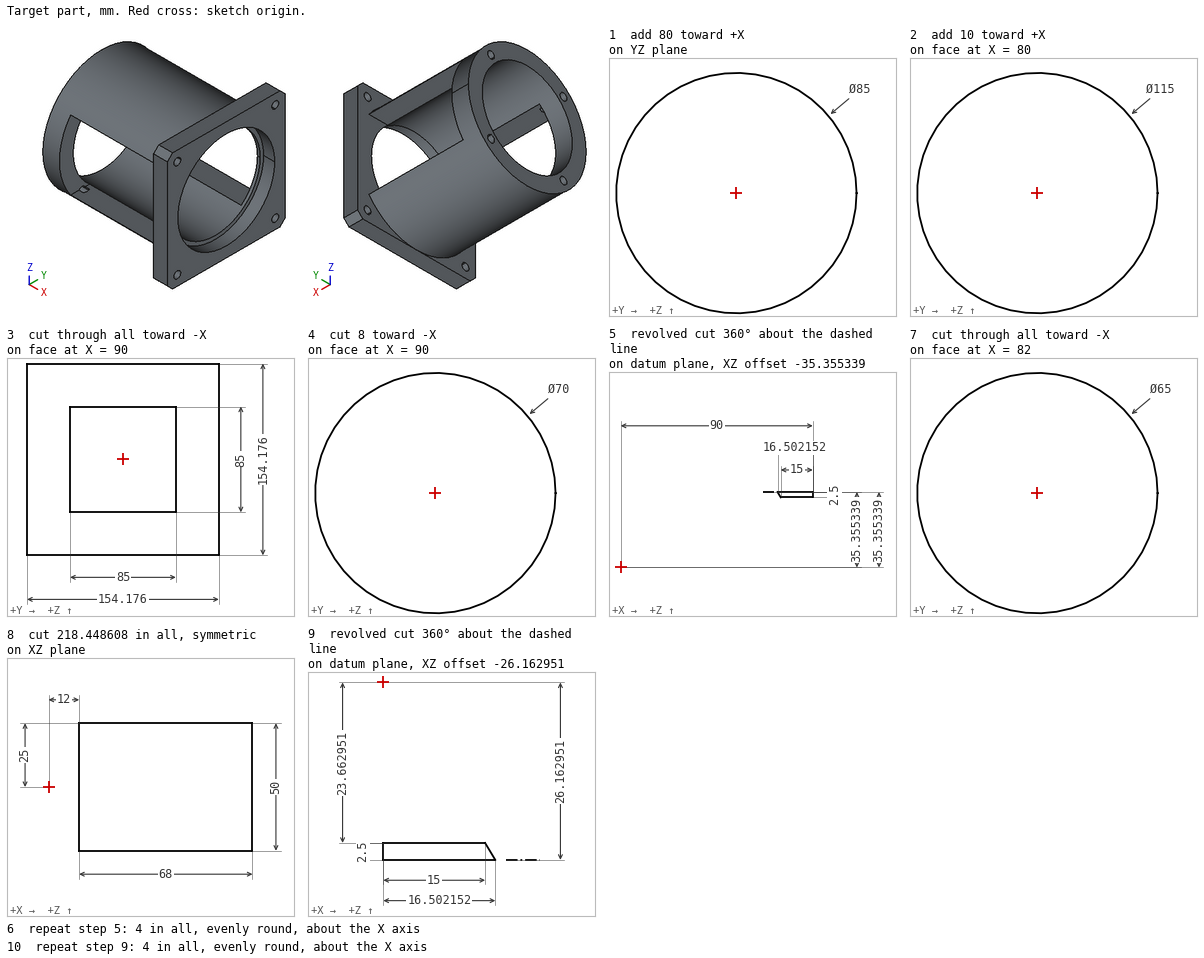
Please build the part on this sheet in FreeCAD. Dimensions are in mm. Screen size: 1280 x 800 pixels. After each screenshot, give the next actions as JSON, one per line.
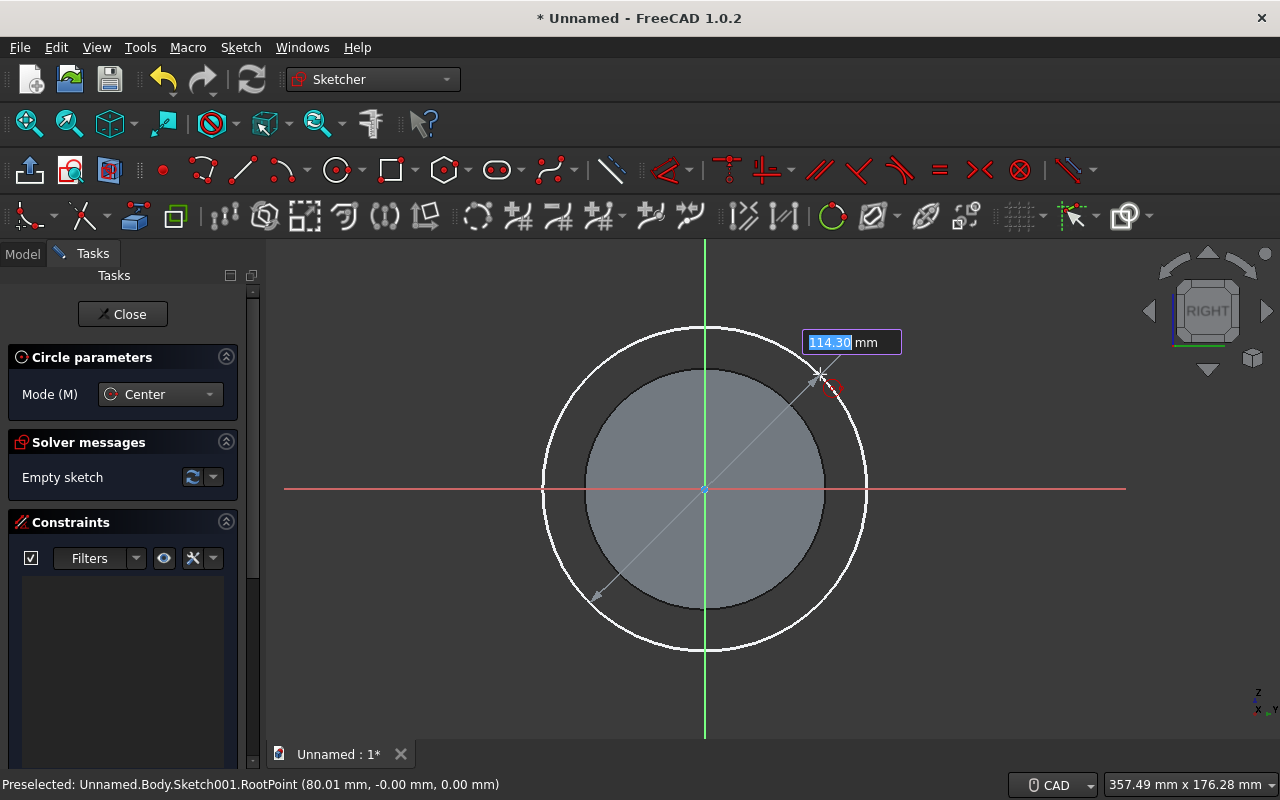
{"action": "type", "text": "115"}
{"action": "key", "text": "Return"}
{"action": "key", "text": "Escape"}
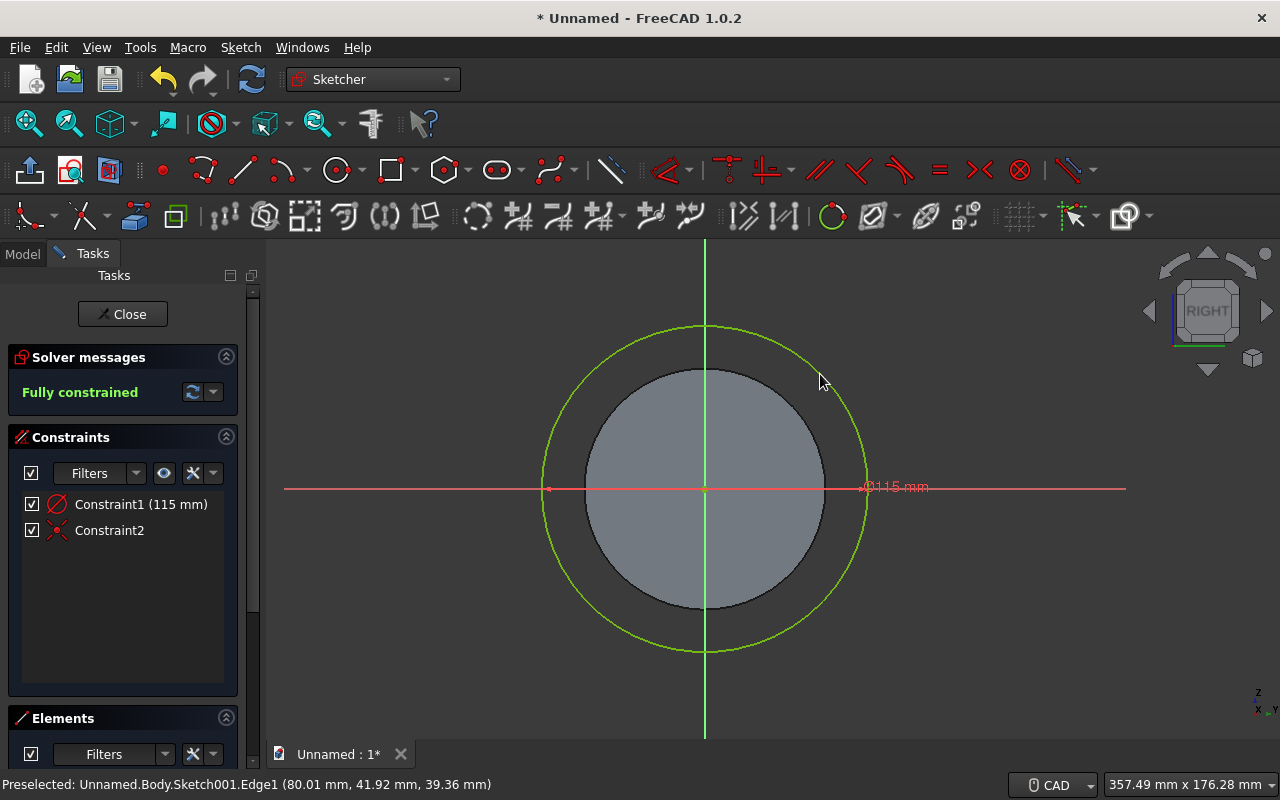
{"action": "left_click", "coordinate": [123, 314]}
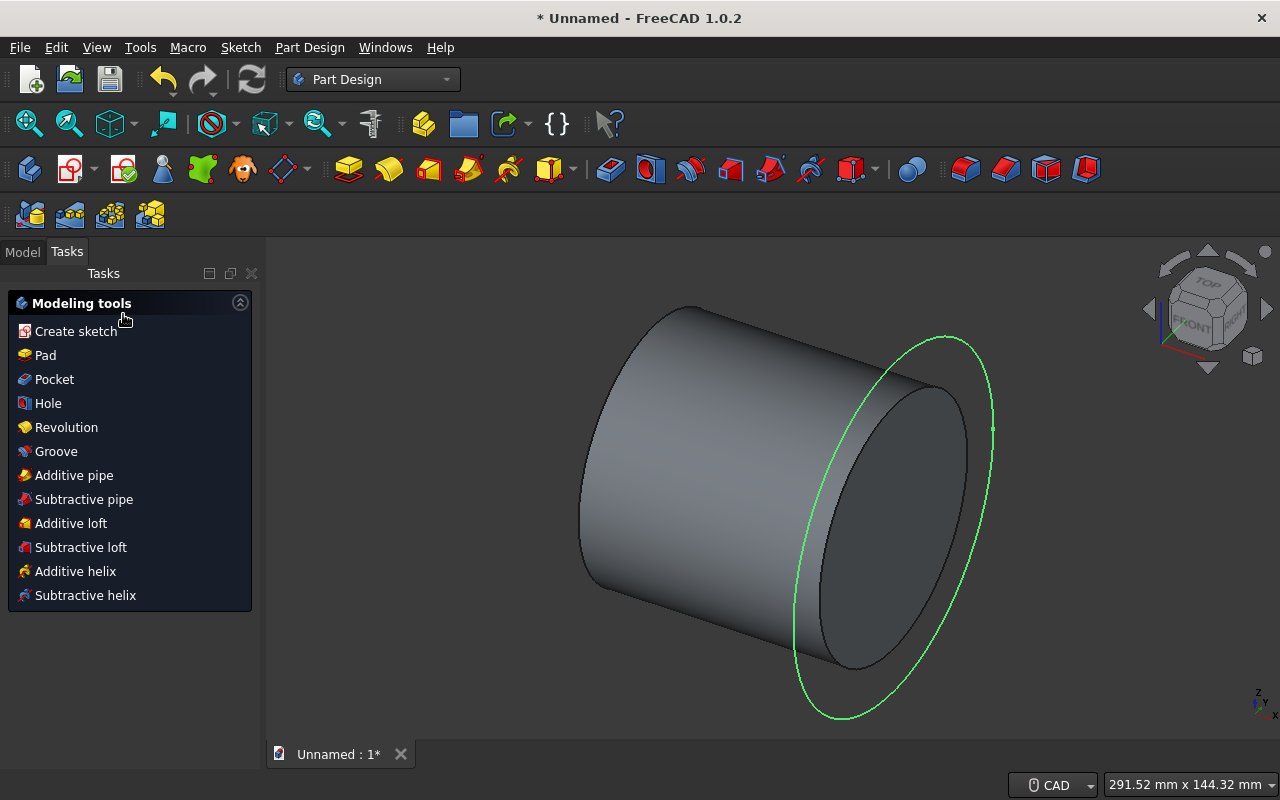
{"action": "left_click", "coordinate": [350, 170]}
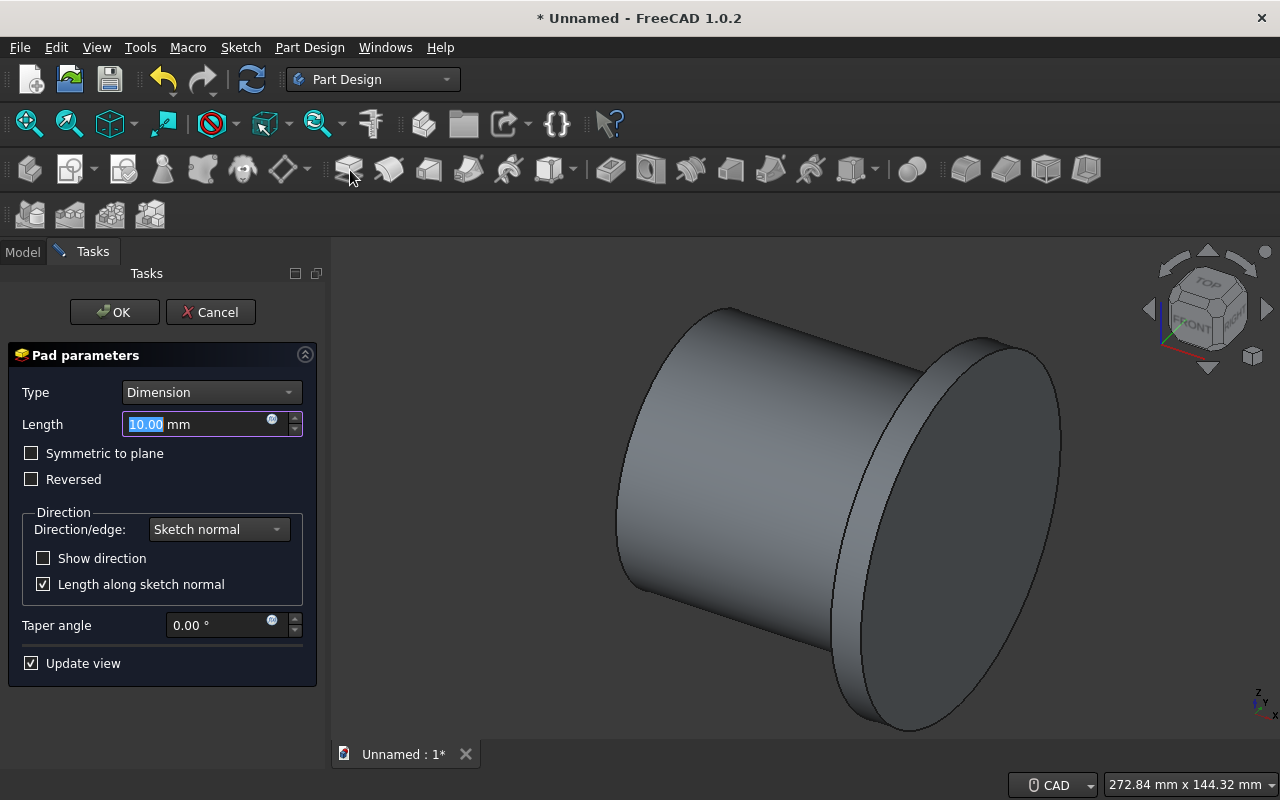
{"action": "type", "text": "10"}
{"action": "key", "text": "Tab"}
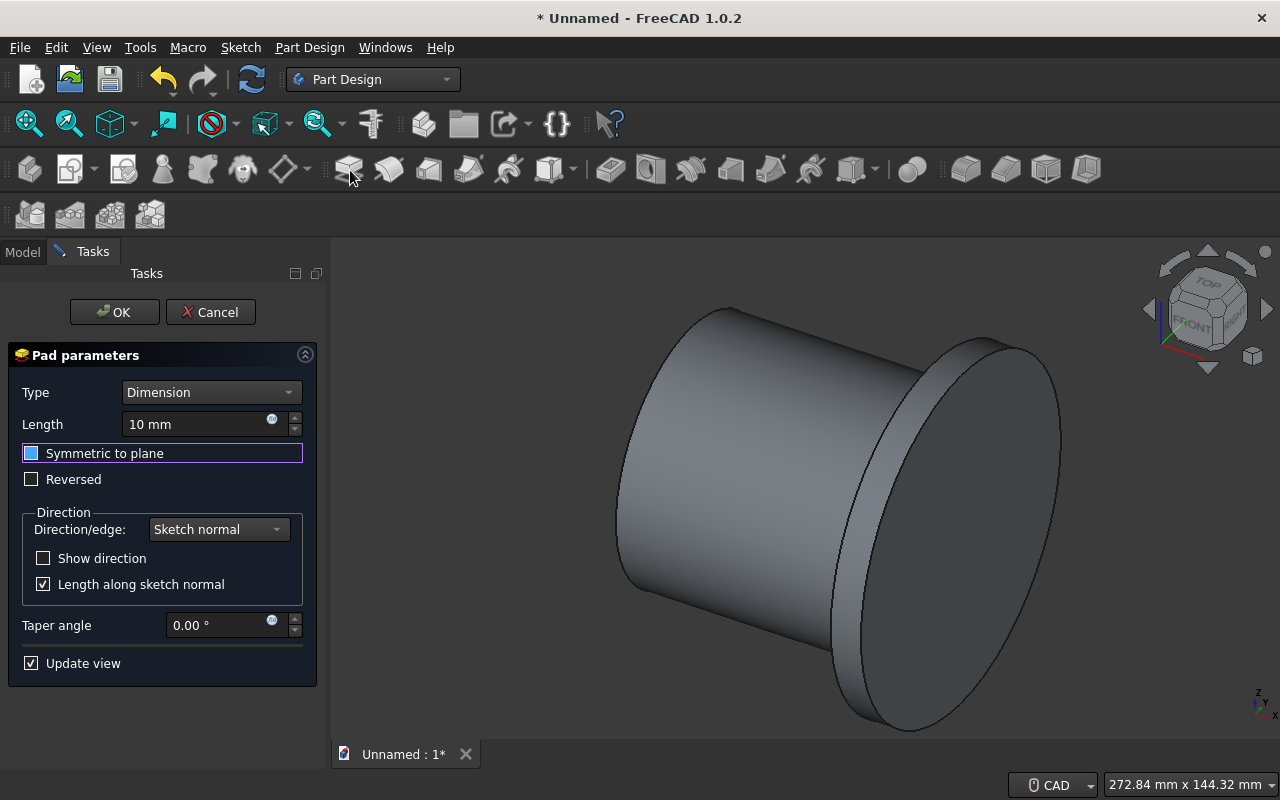
{"action": "left_click", "coordinate": [115, 312]}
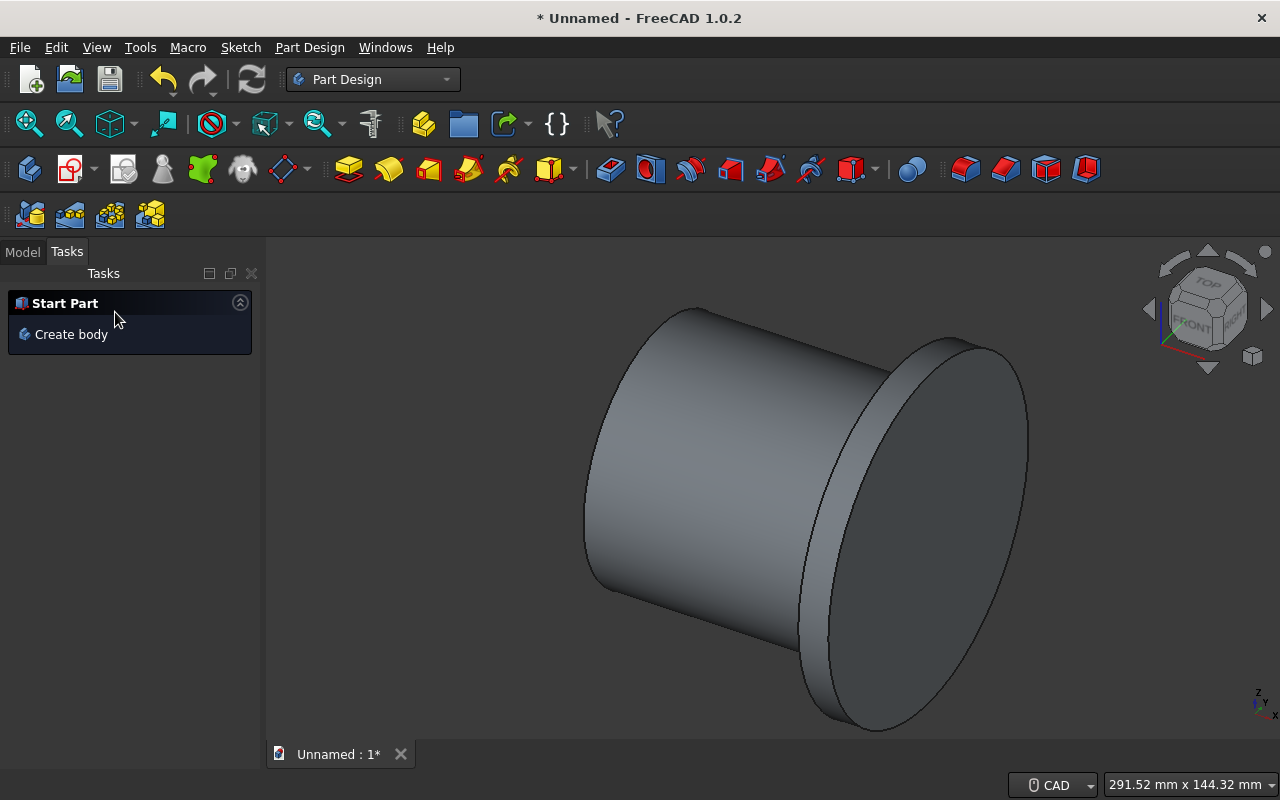
{"action": "left_click", "coordinate": [30, 124]}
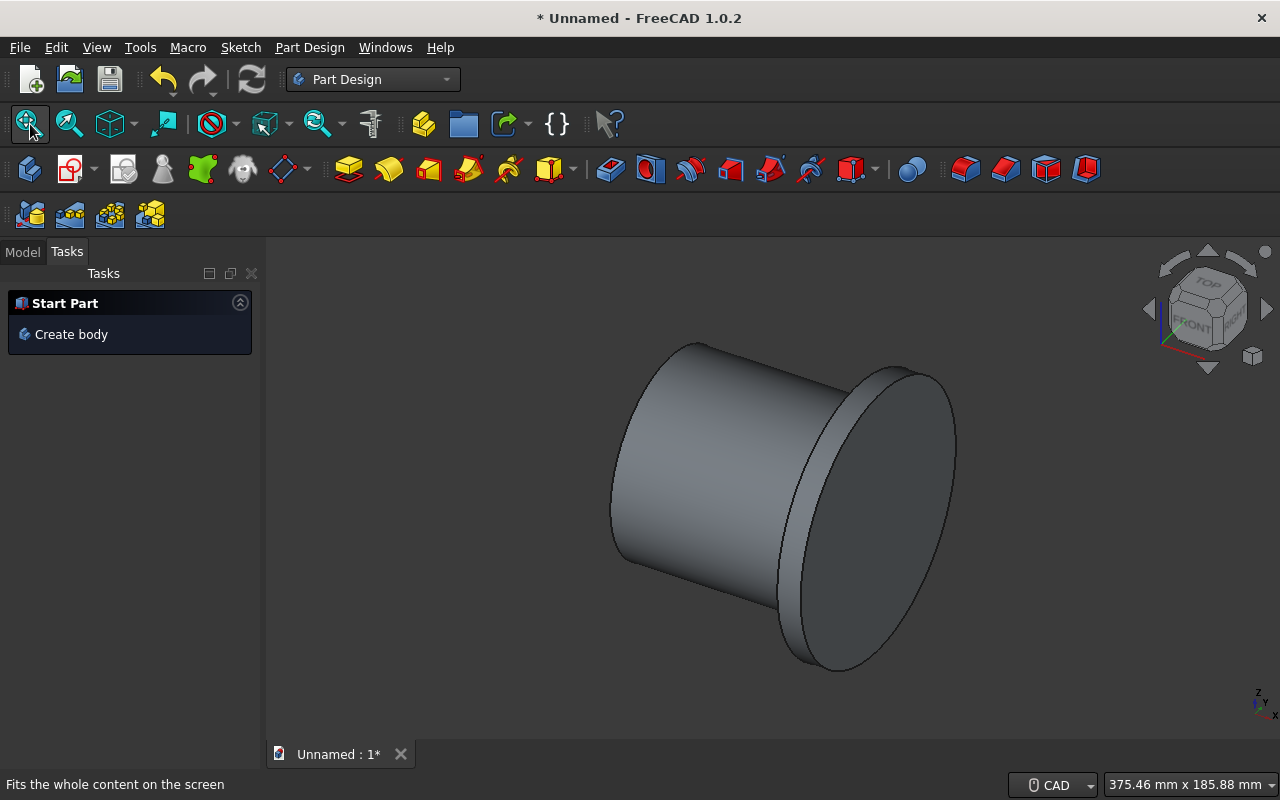
{"action": "left_click", "coordinate": [878, 522]}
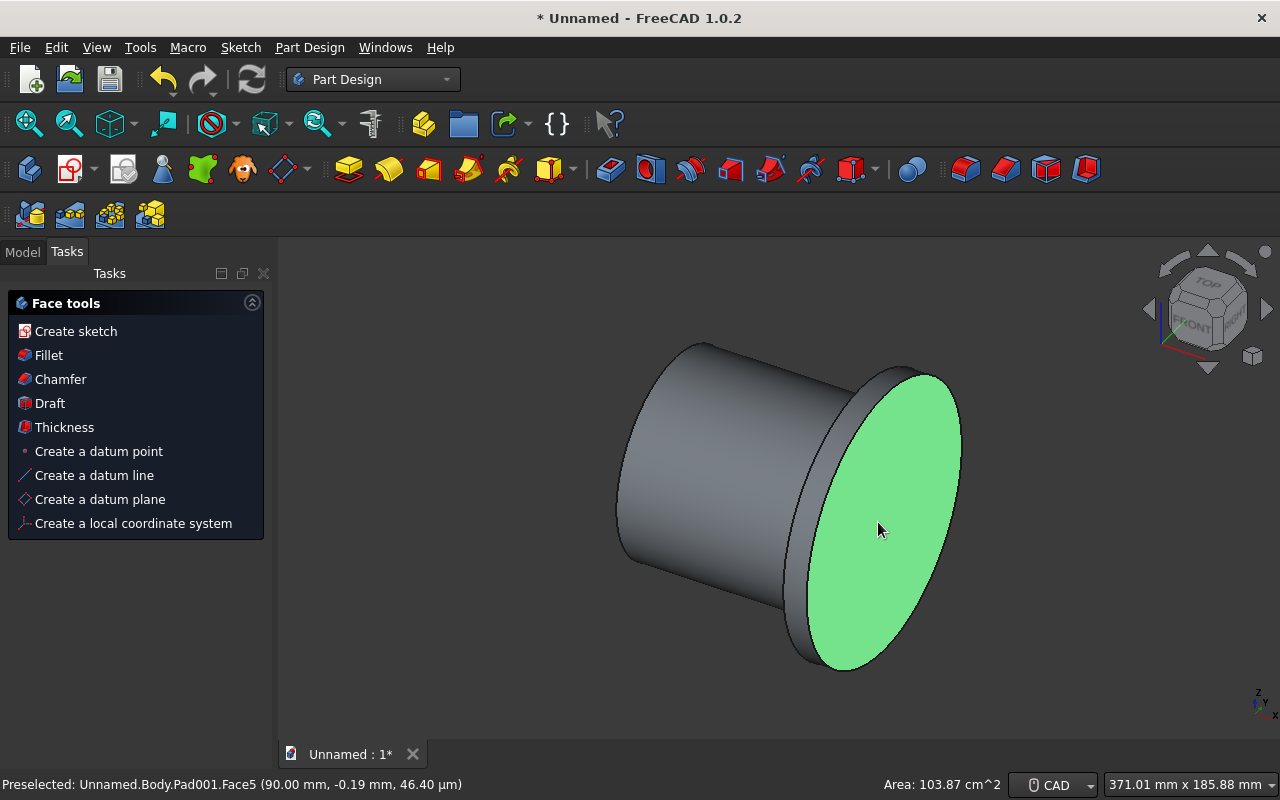
{"action": "left_click", "coordinate": [70, 170]}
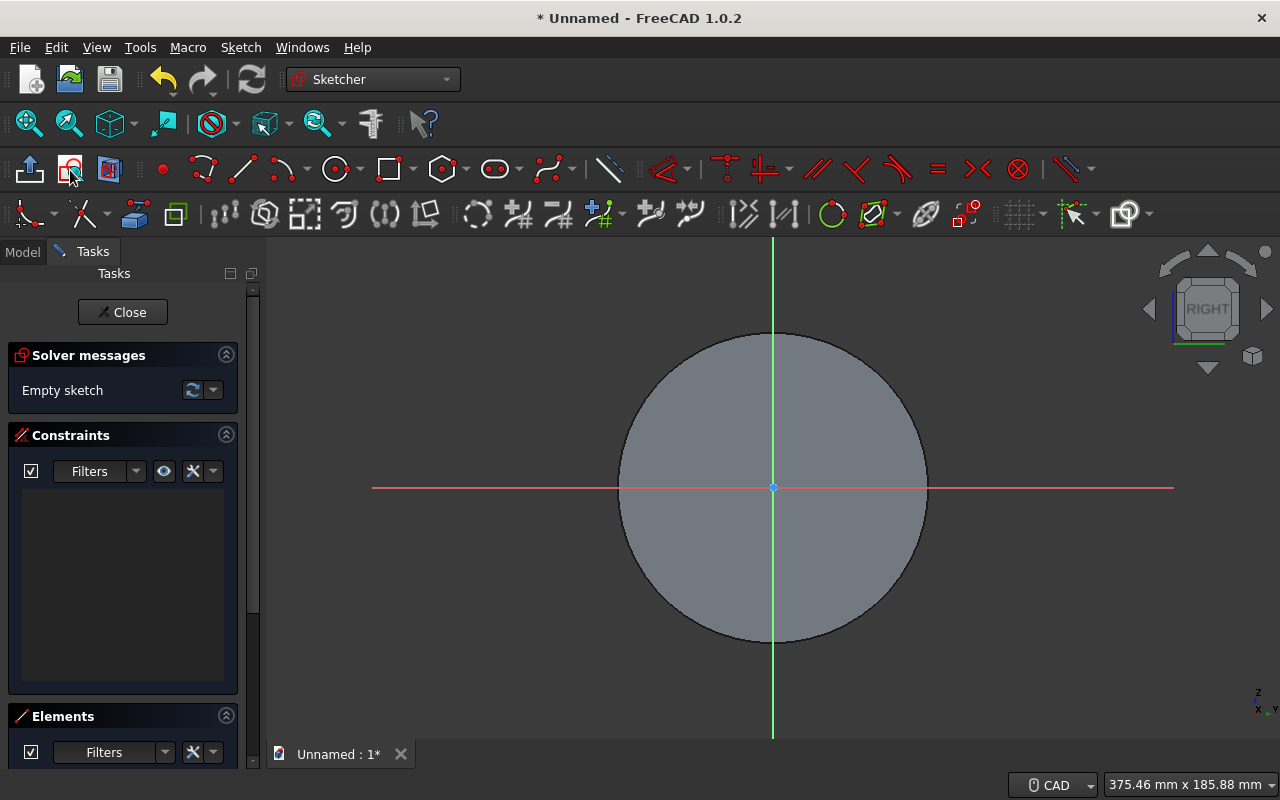
{"action": "scroll", "coordinate": [395, 488], "scroll_direction": "down", "scroll_amount": 1}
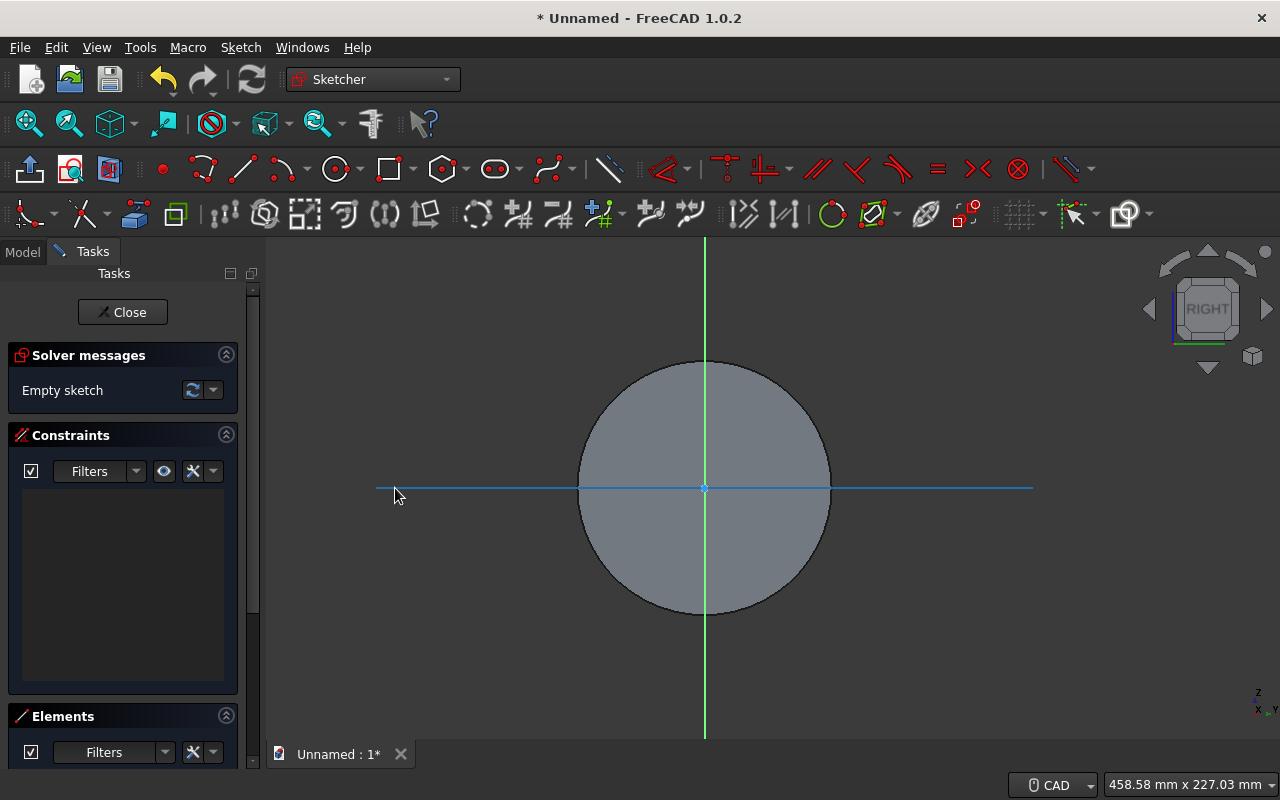
{"action": "key", "text": "g v"}